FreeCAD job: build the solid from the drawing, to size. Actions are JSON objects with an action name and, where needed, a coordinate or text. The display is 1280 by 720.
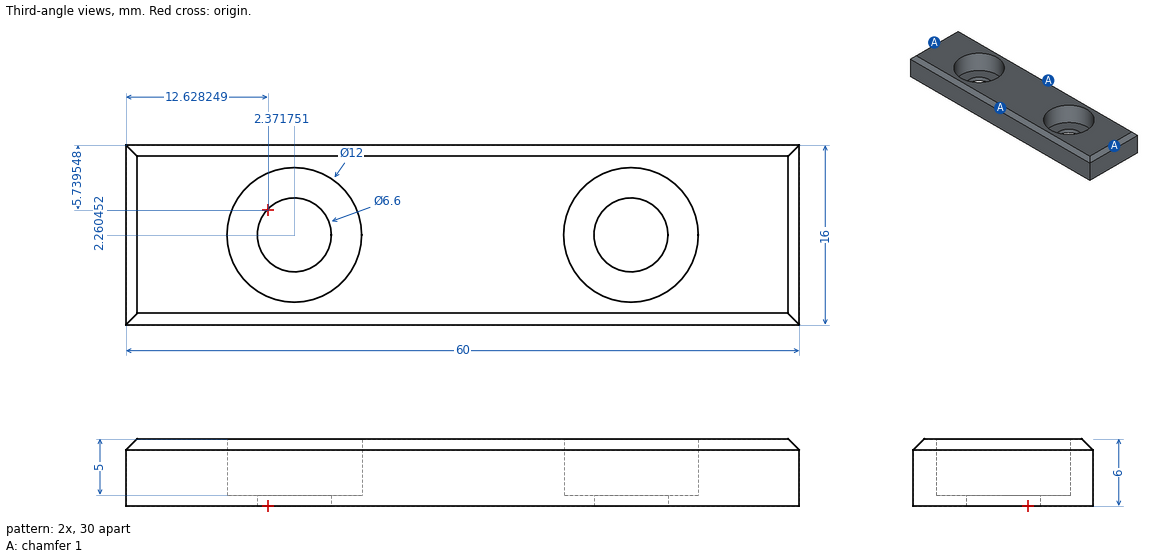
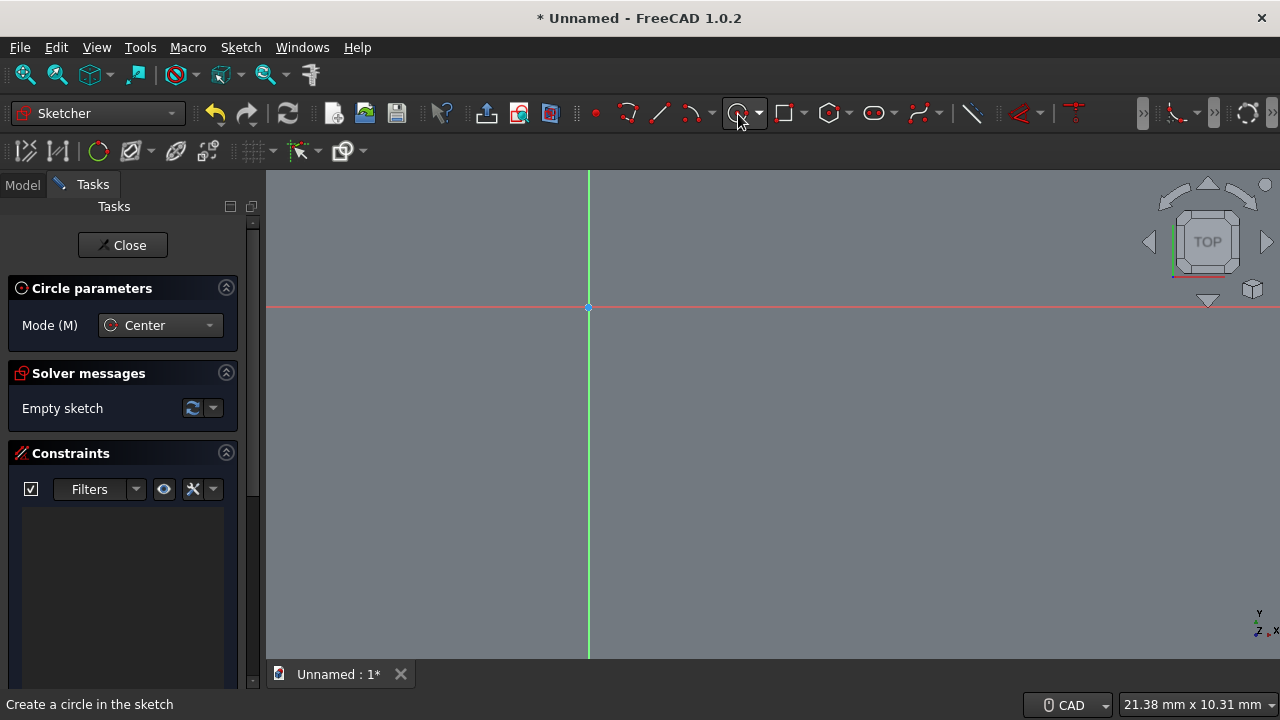
{"action": "left_click", "coordinate": [701, 414]}
{"action": "mouse_move", "coordinate": [812, 525]}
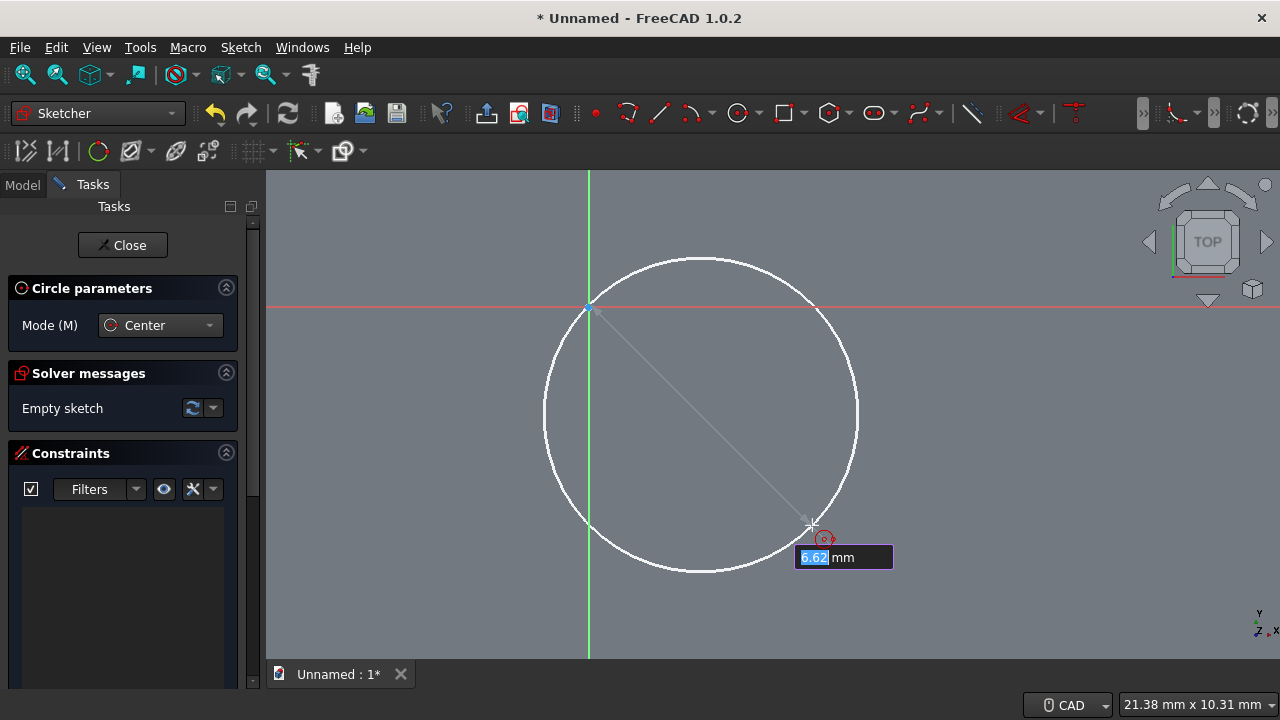
{"action": "type", "text": "6.6"}
{"action": "key", "text": "Return"}
{"action": "key", "text": "Escape"}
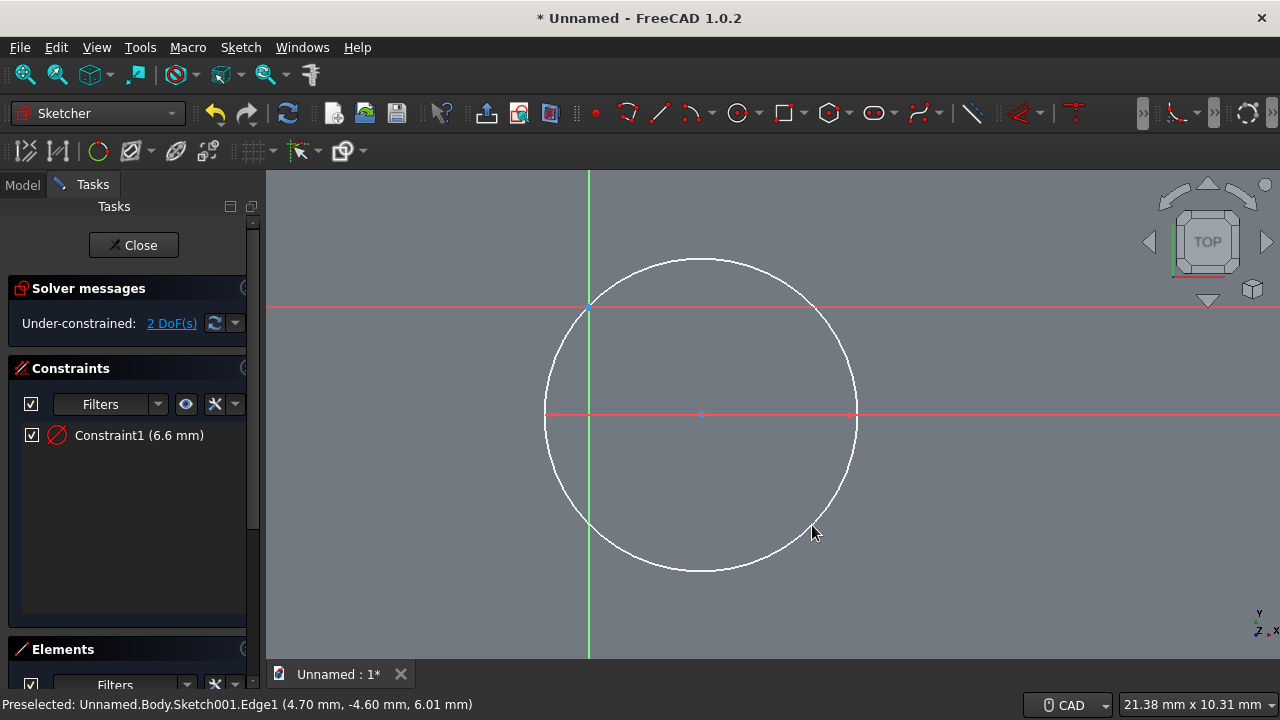
{"action": "left_click", "coordinate": [1020, 114]}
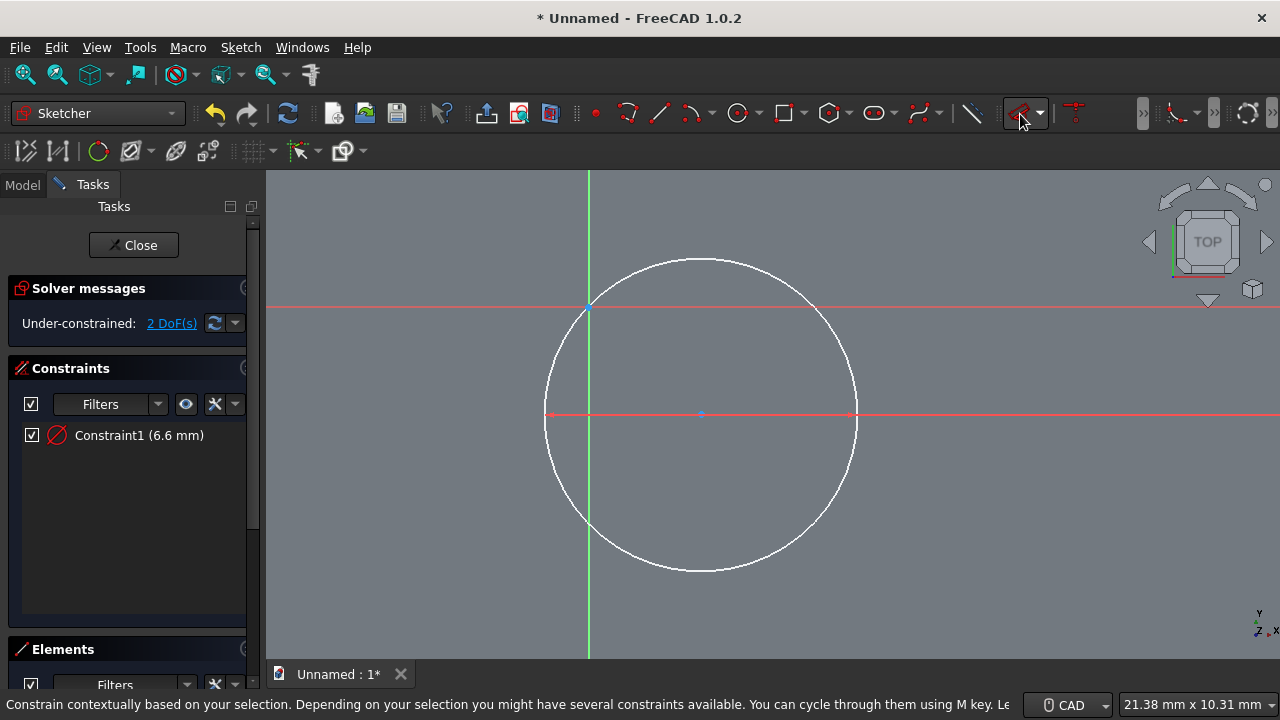
{"action": "left_click", "coordinate": [701, 415]}
{"action": "left_click", "coordinate": [606, 273]}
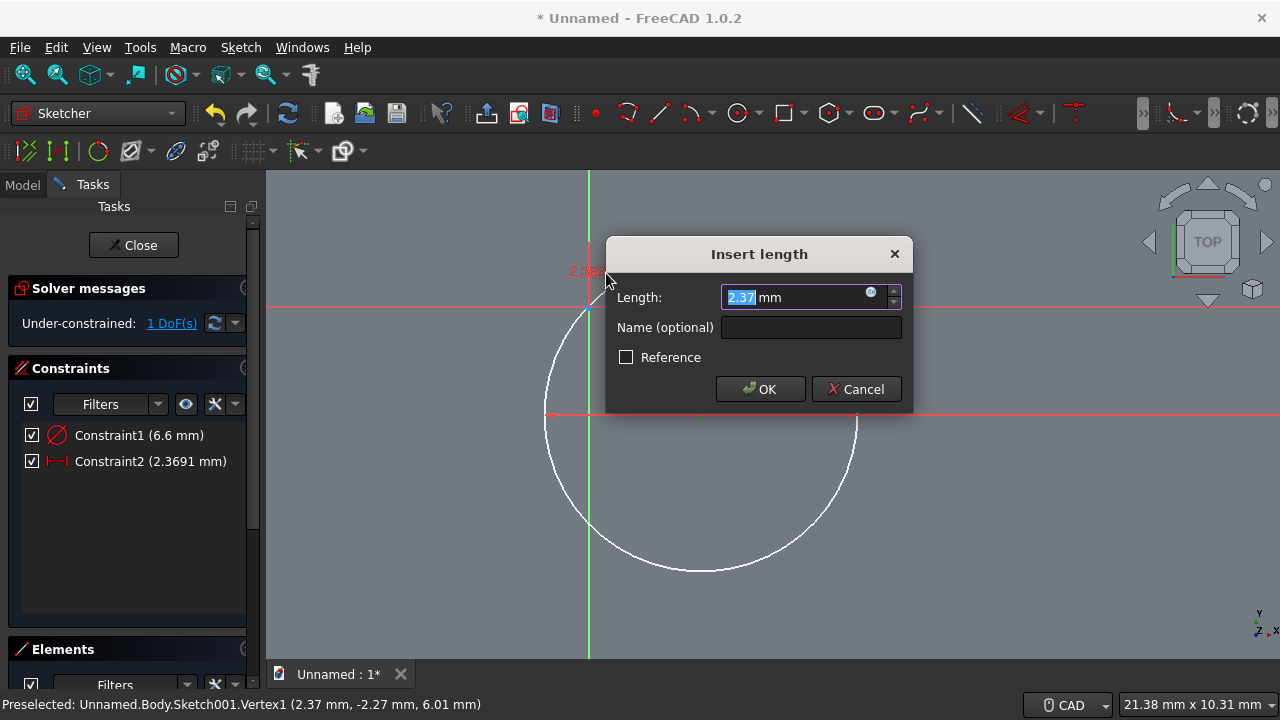
{"action": "type", "text": "2.371751"}
{"action": "key", "text": "Return"}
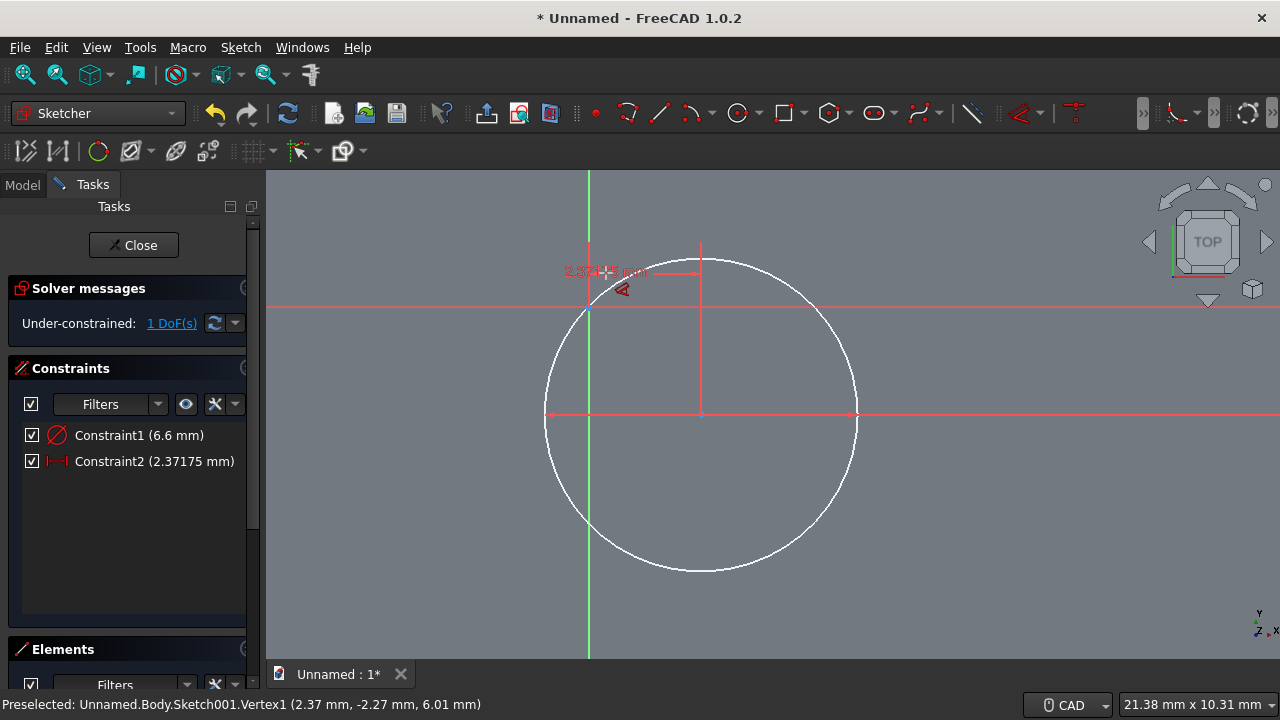
{"action": "left_click", "coordinate": [701, 415]}
{"action": "left_click", "coordinate": [555, 323]}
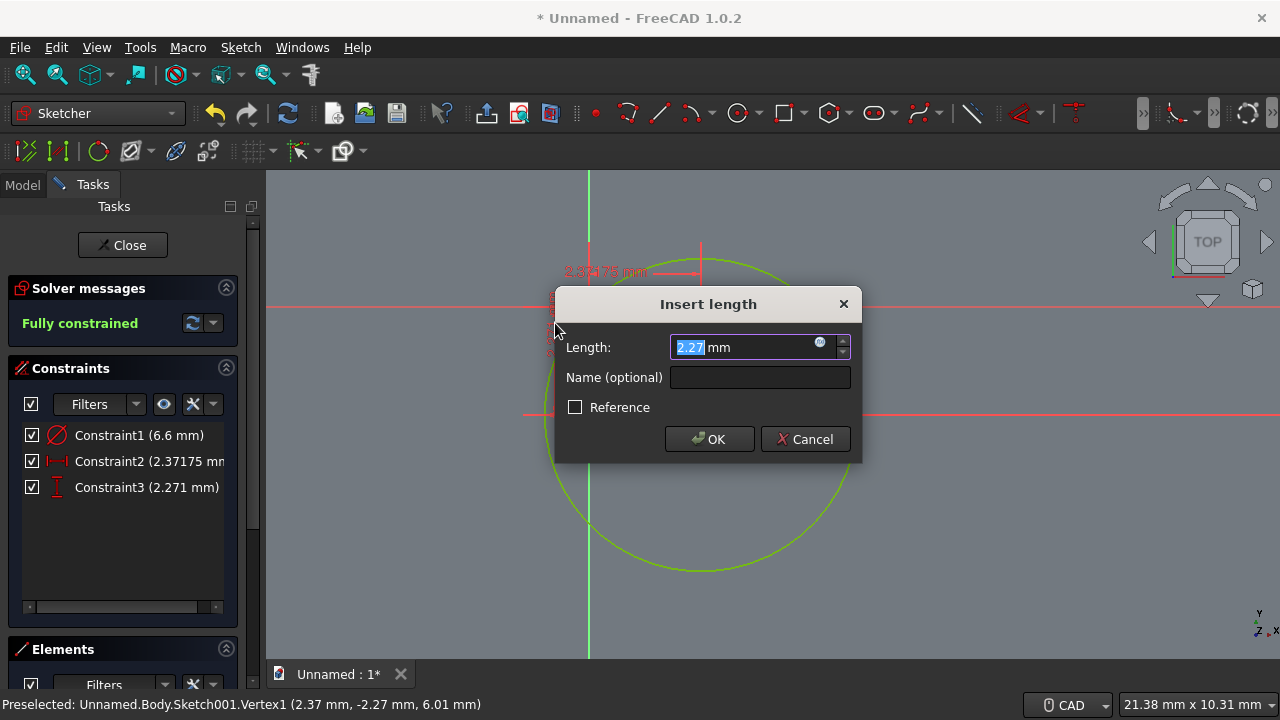
{"action": "type", "text": "2.260452"}
{"action": "key", "text": "Return"}
{"action": "key", "text": "Escape"}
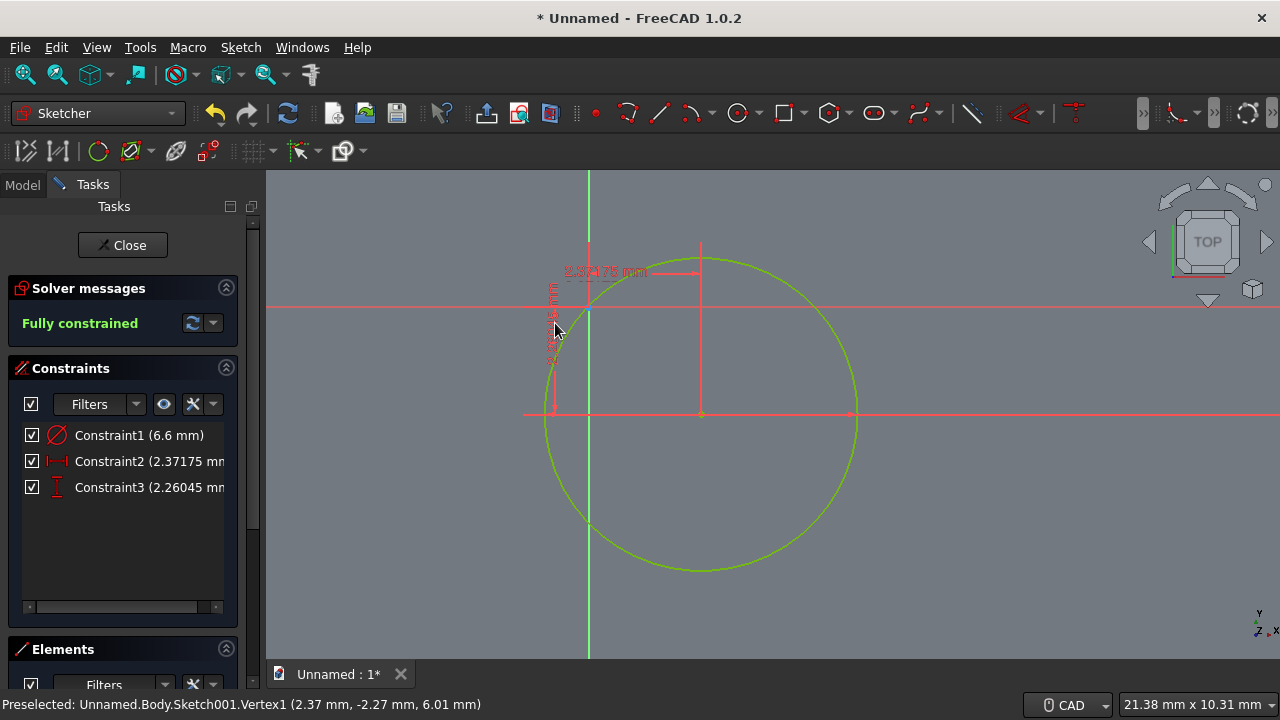
{"action": "left_click", "coordinate": [123, 245]}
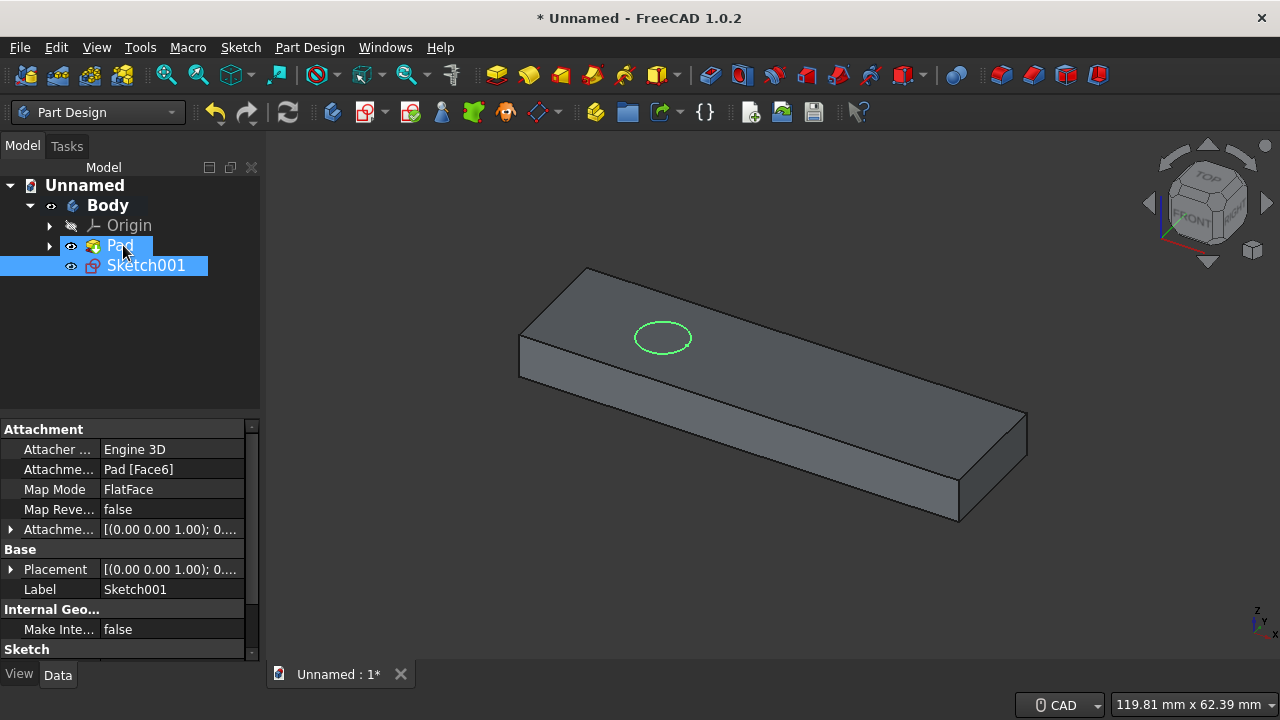
{"action": "left_click", "coordinate": [712, 76]}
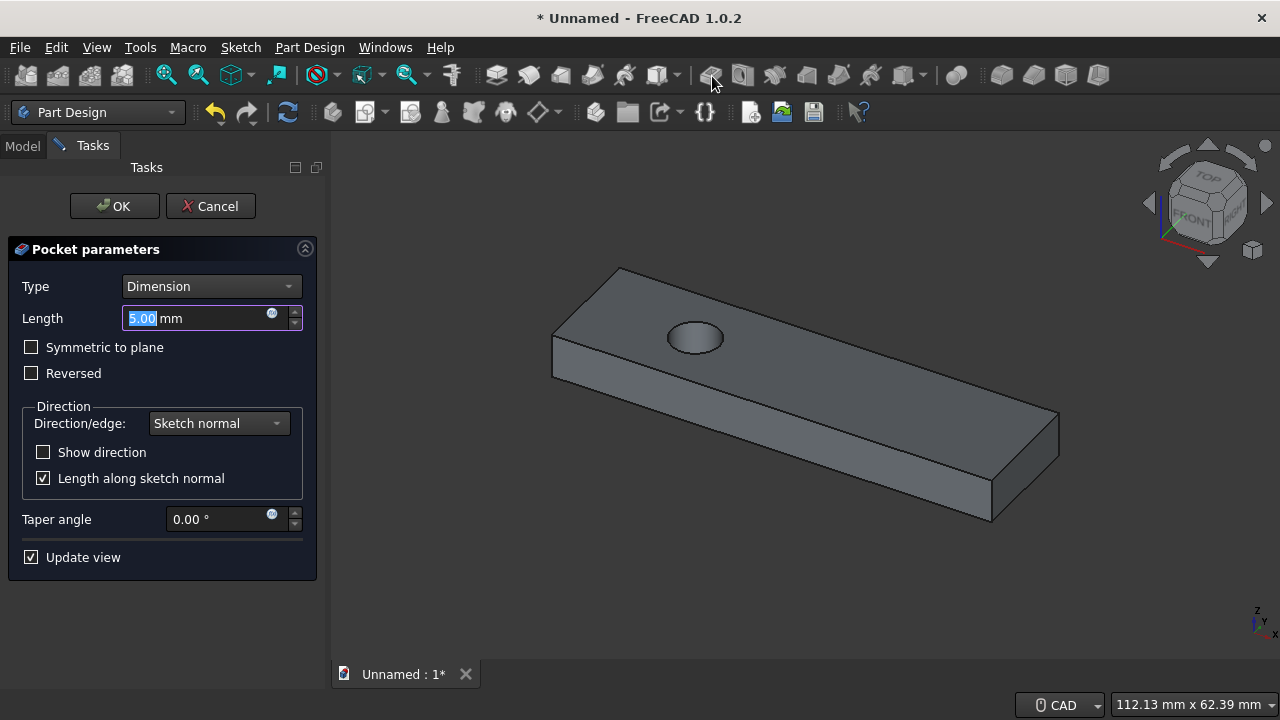
{"action": "left_click", "coordinate": [212, 286]}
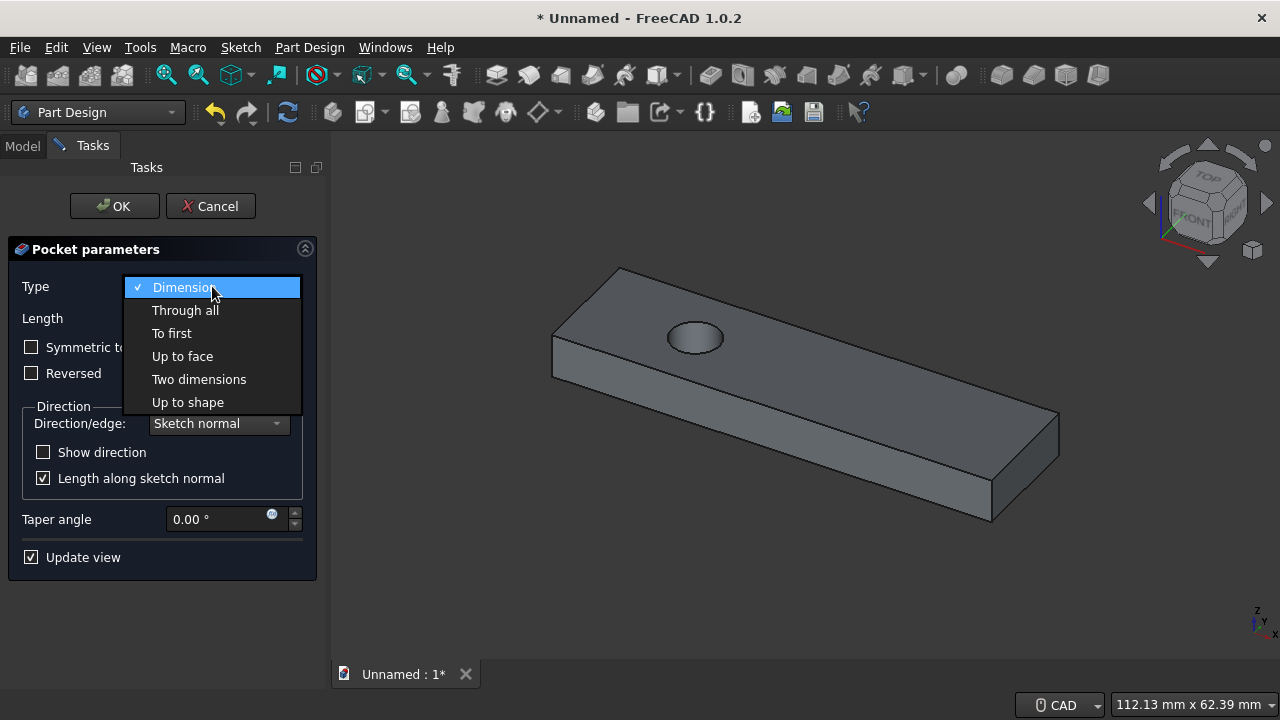
{"action": "left_click", "coordinate": [212, 310]}